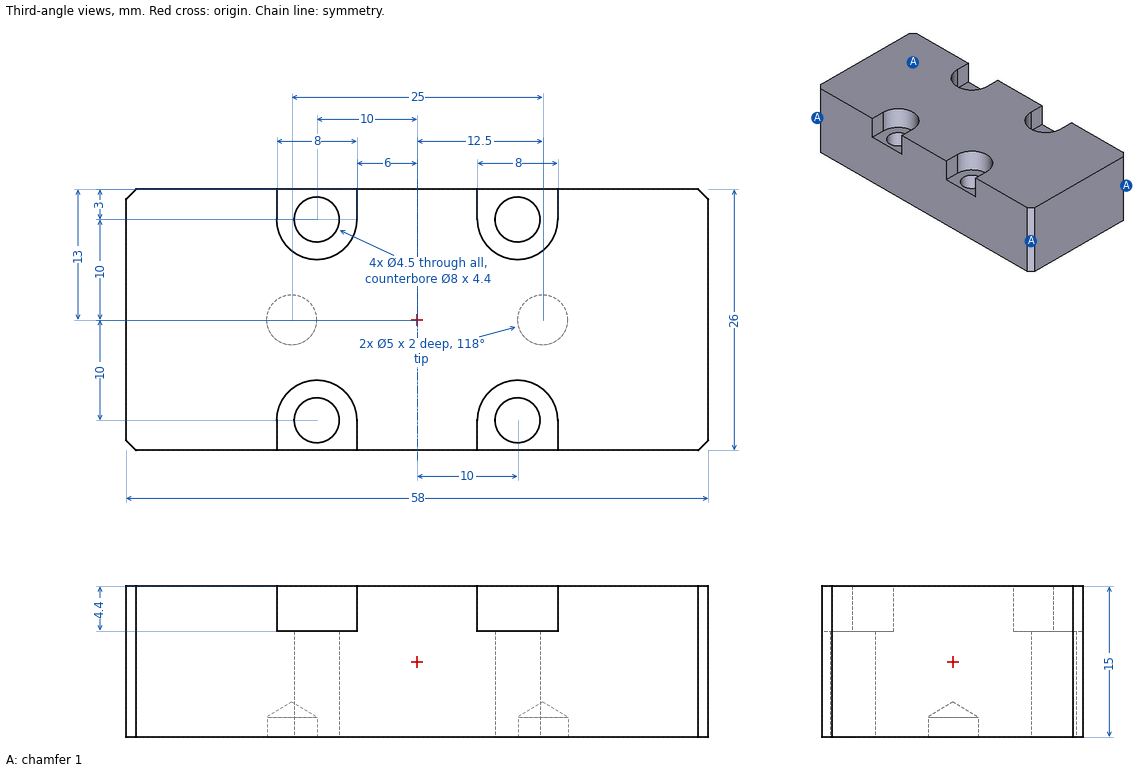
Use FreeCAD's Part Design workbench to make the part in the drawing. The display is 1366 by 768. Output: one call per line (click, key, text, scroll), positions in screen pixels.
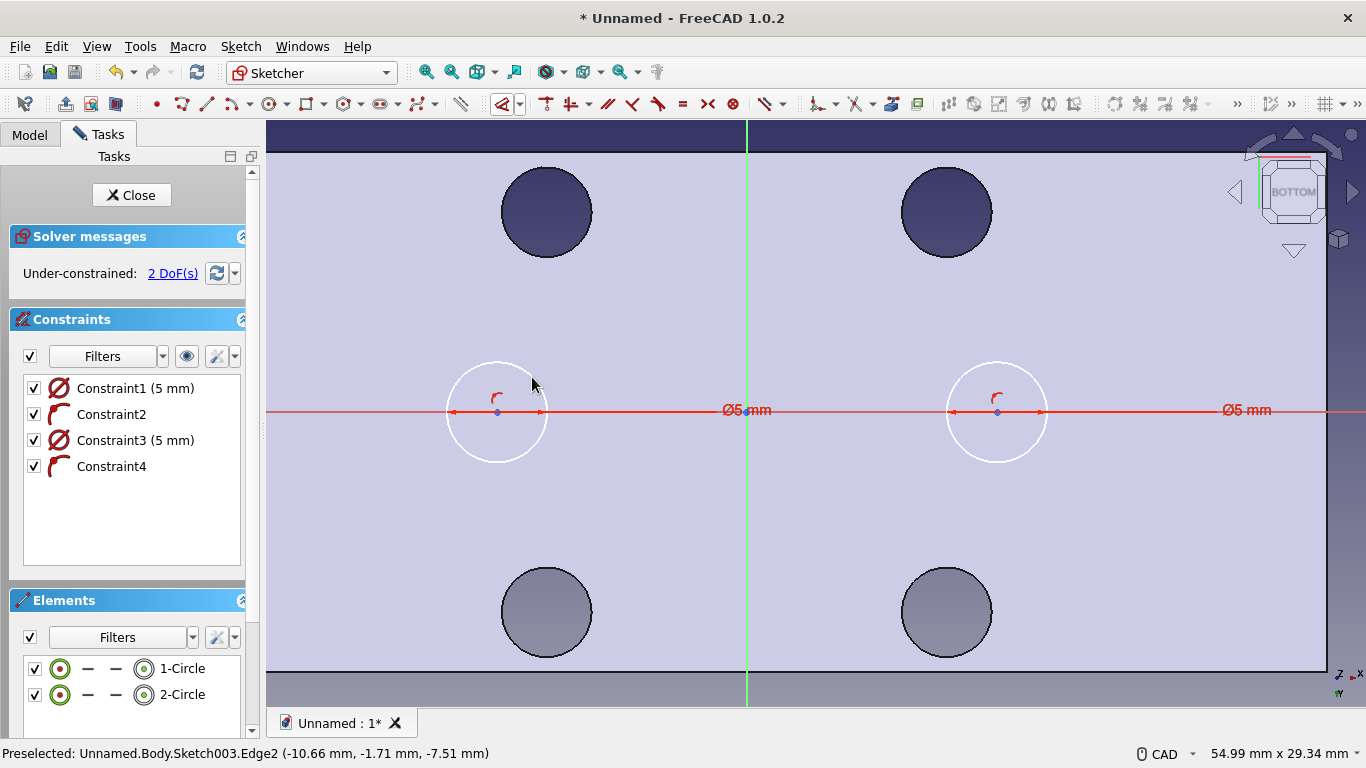
click(997, 412)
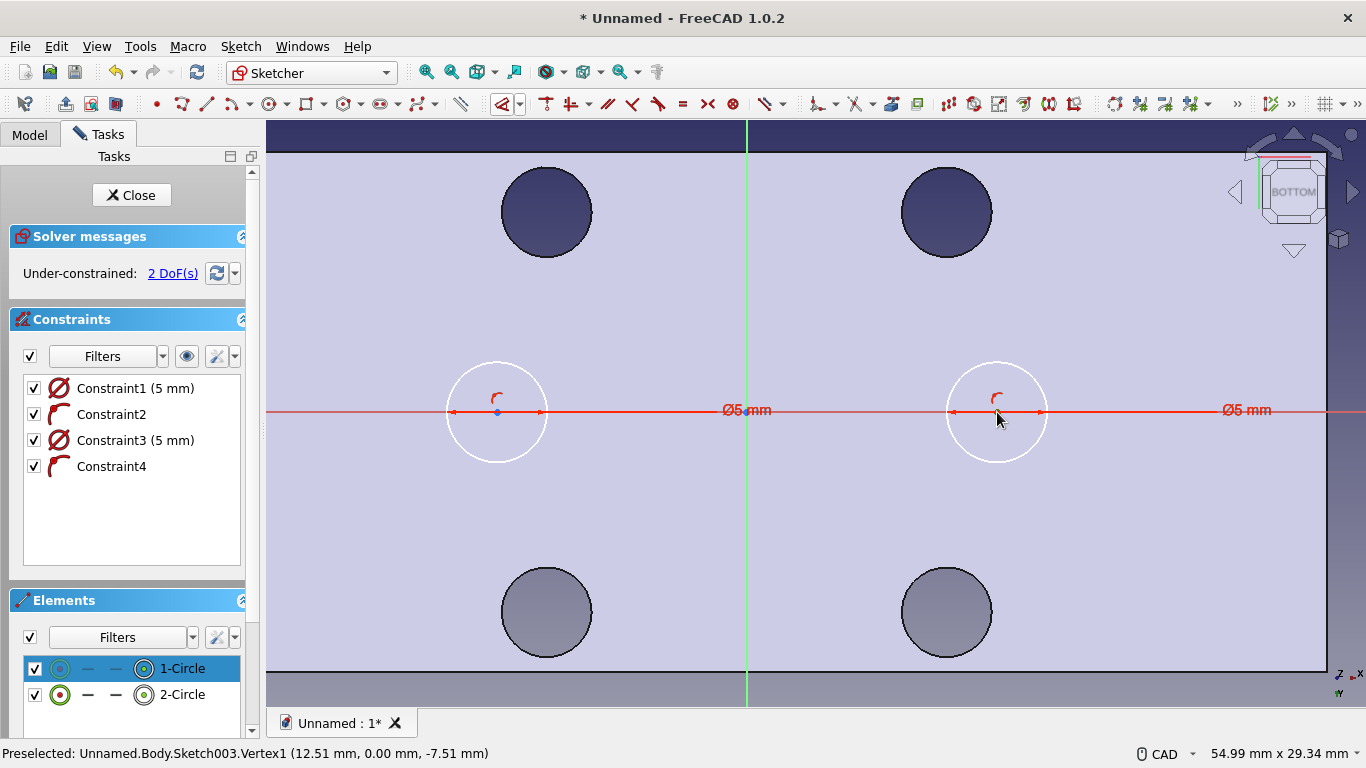
click(497, 412)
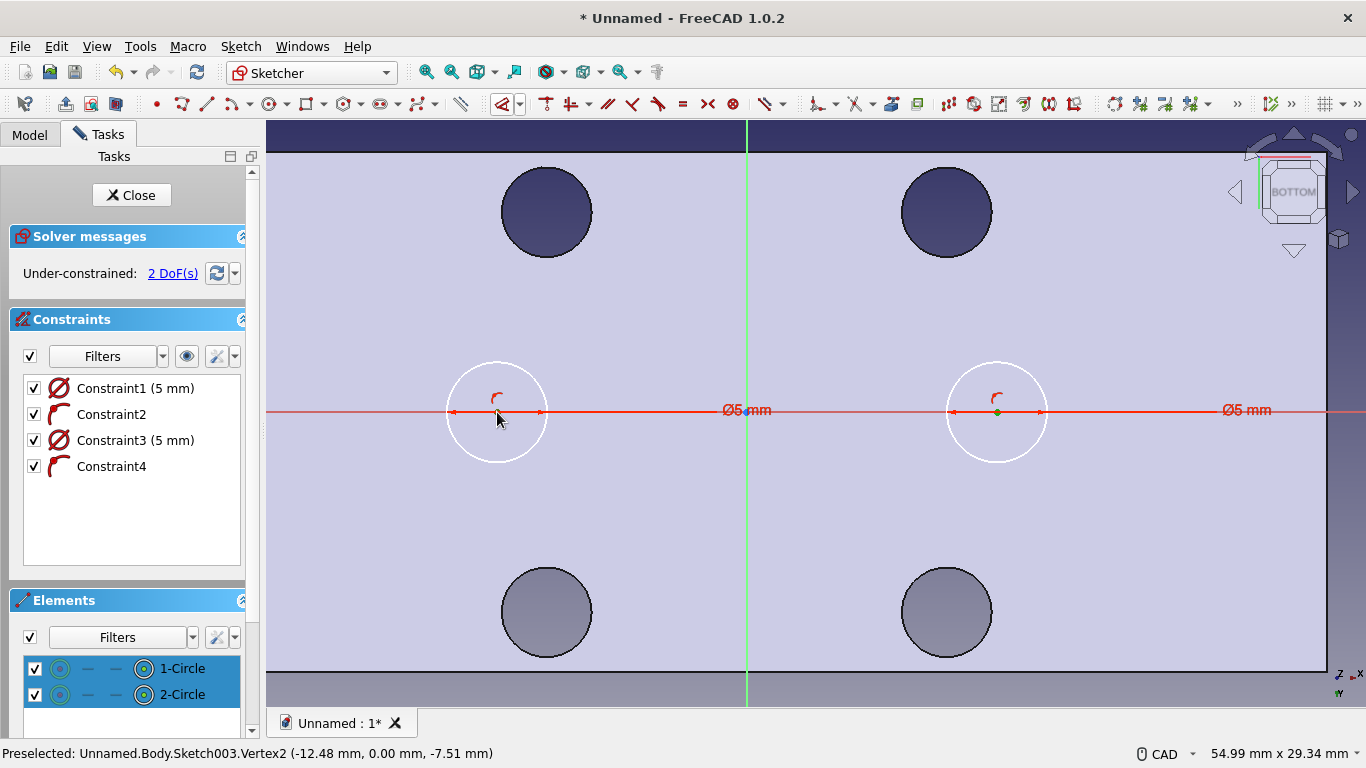
click(520, 104)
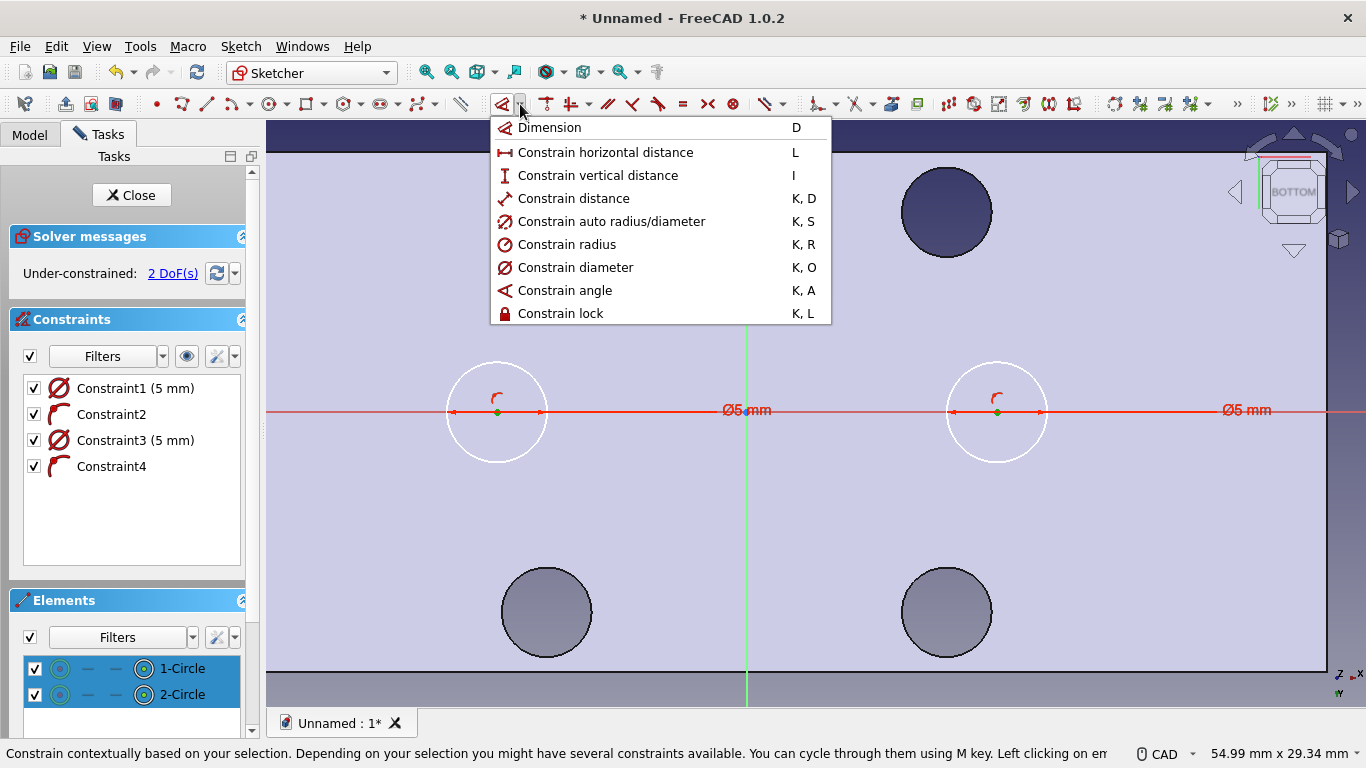
click(661, 152)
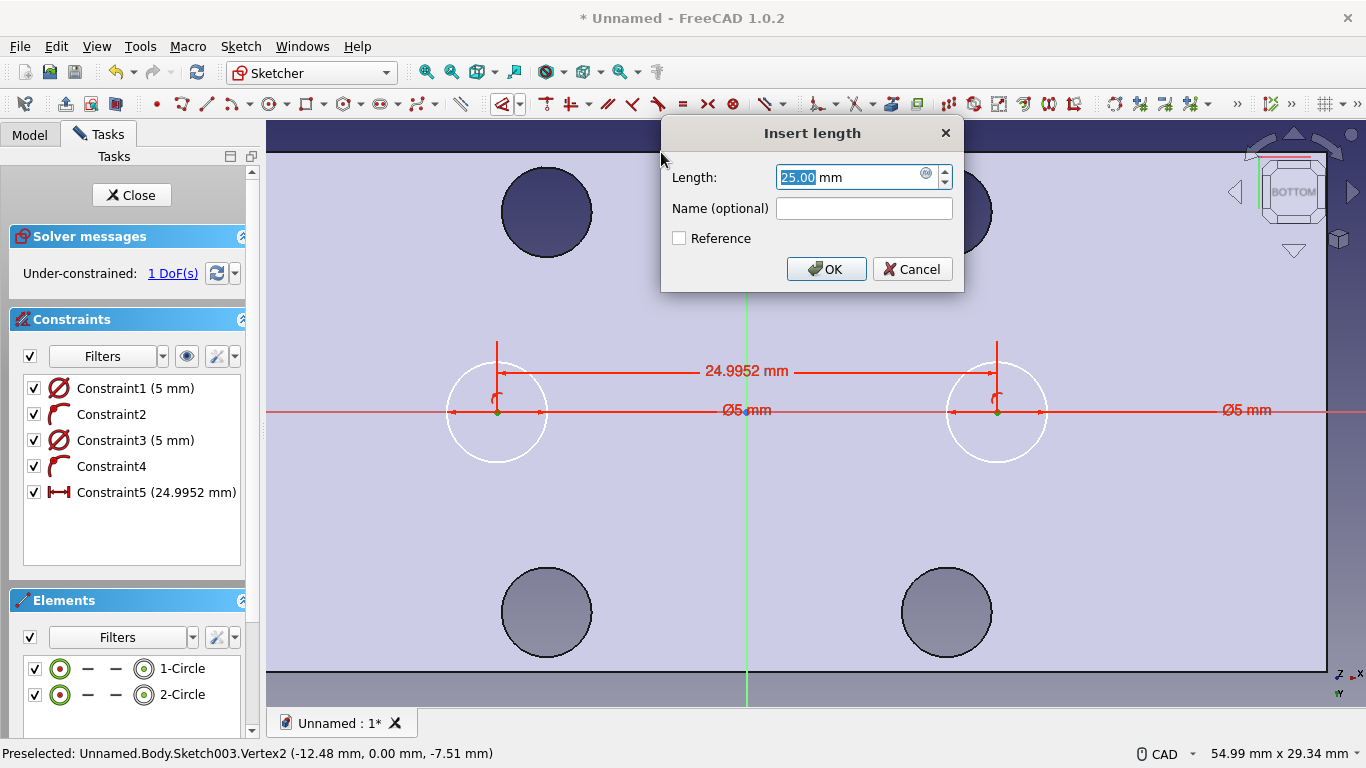
text(25)
key(Return)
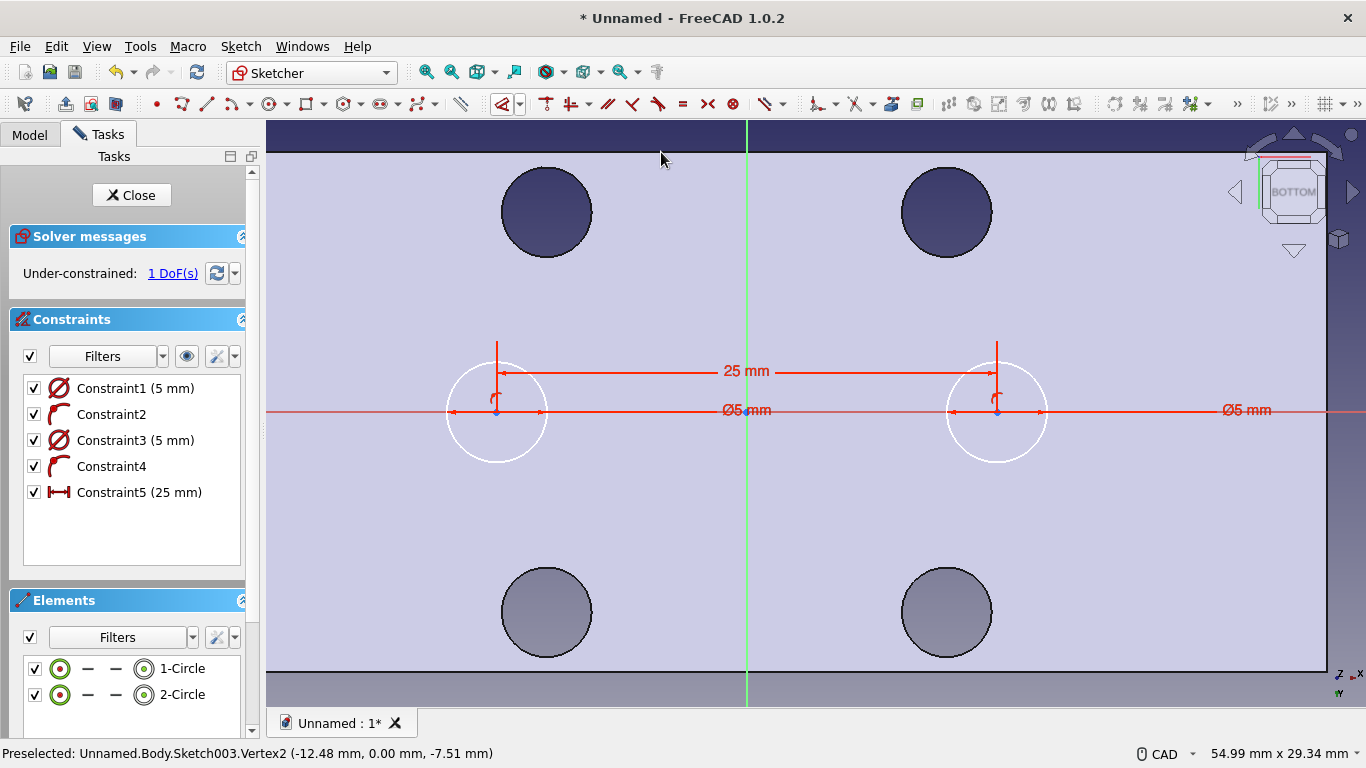
click(997, 412)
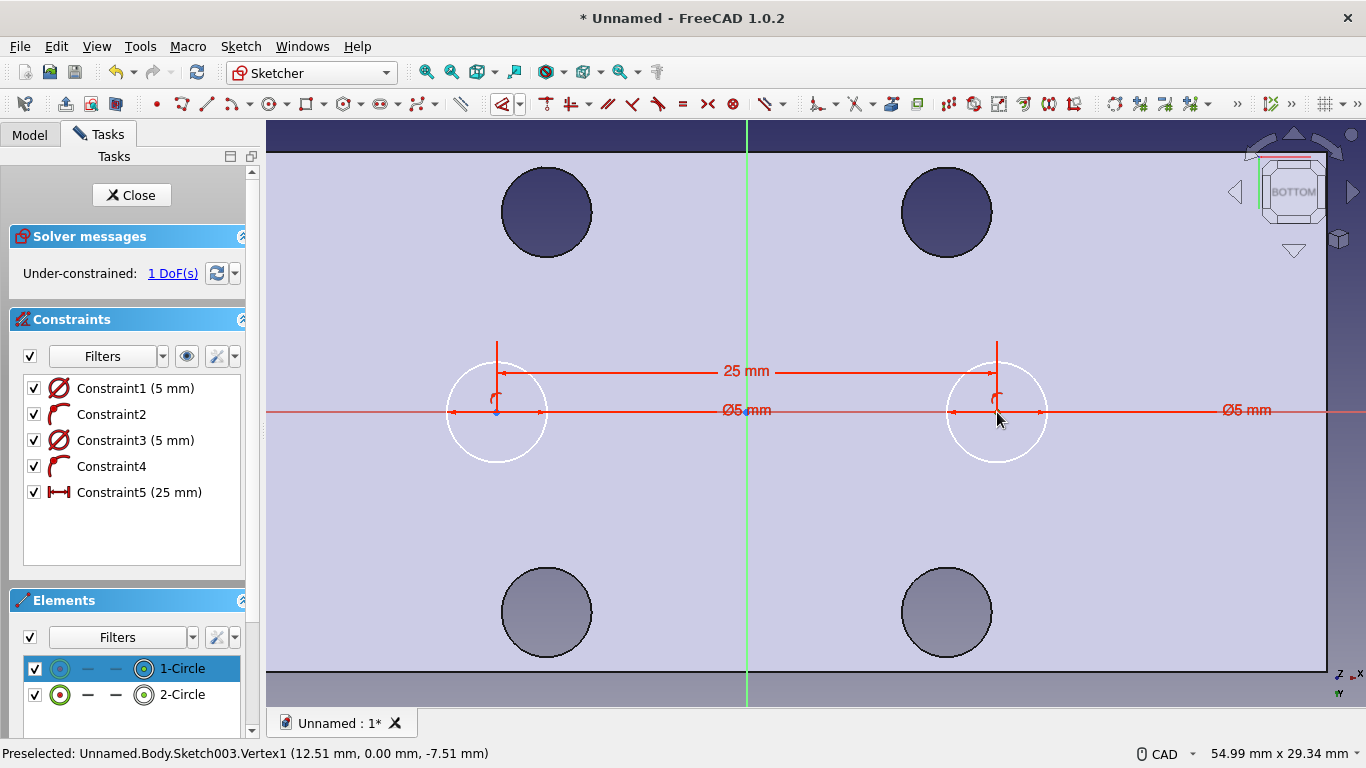
key(l)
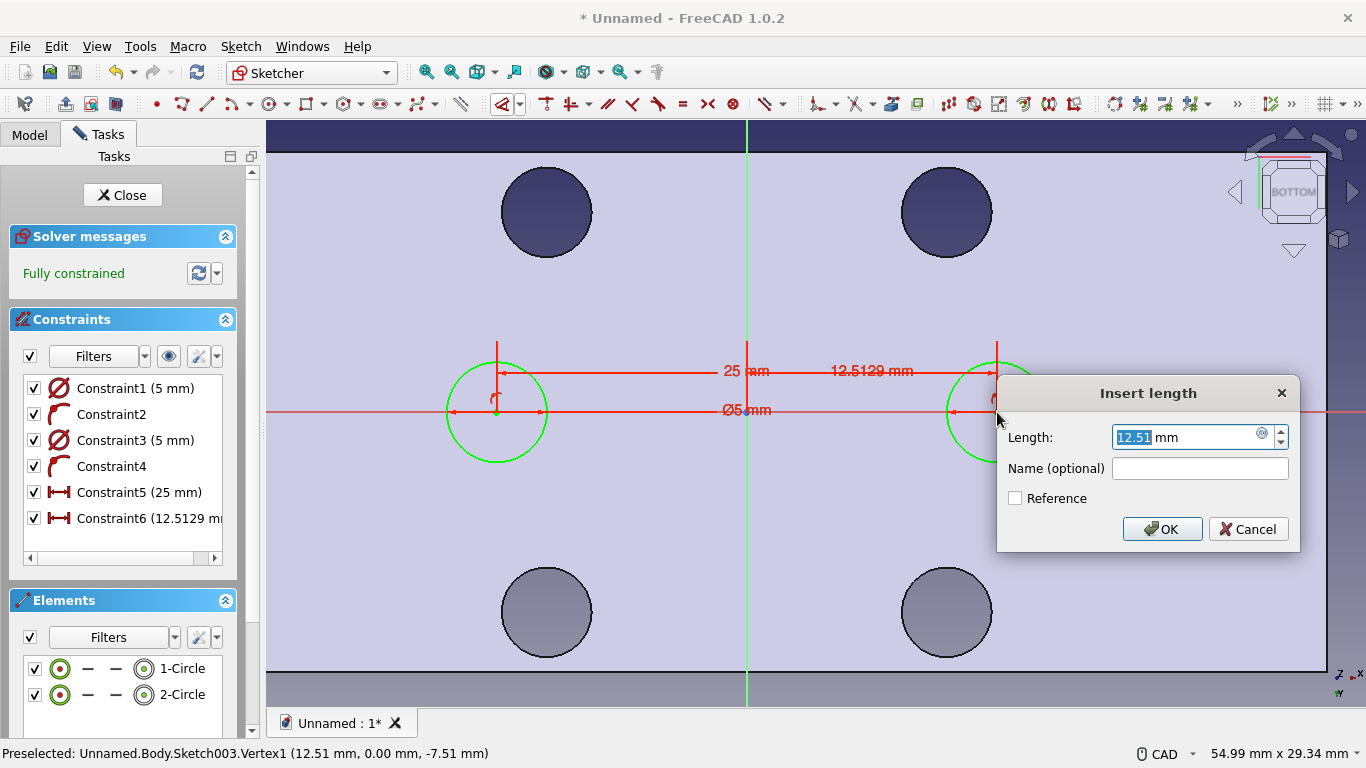
text(12.5)
key(Return)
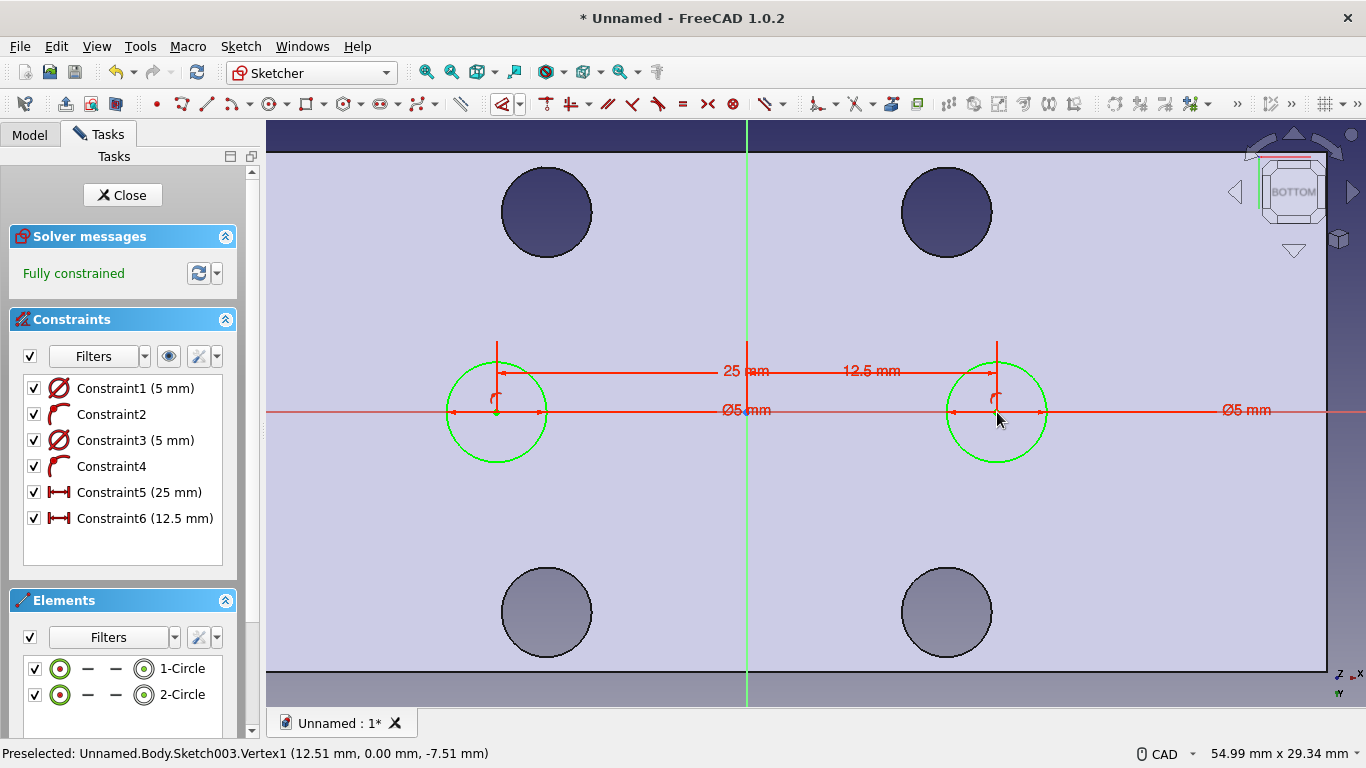
click(123, 195)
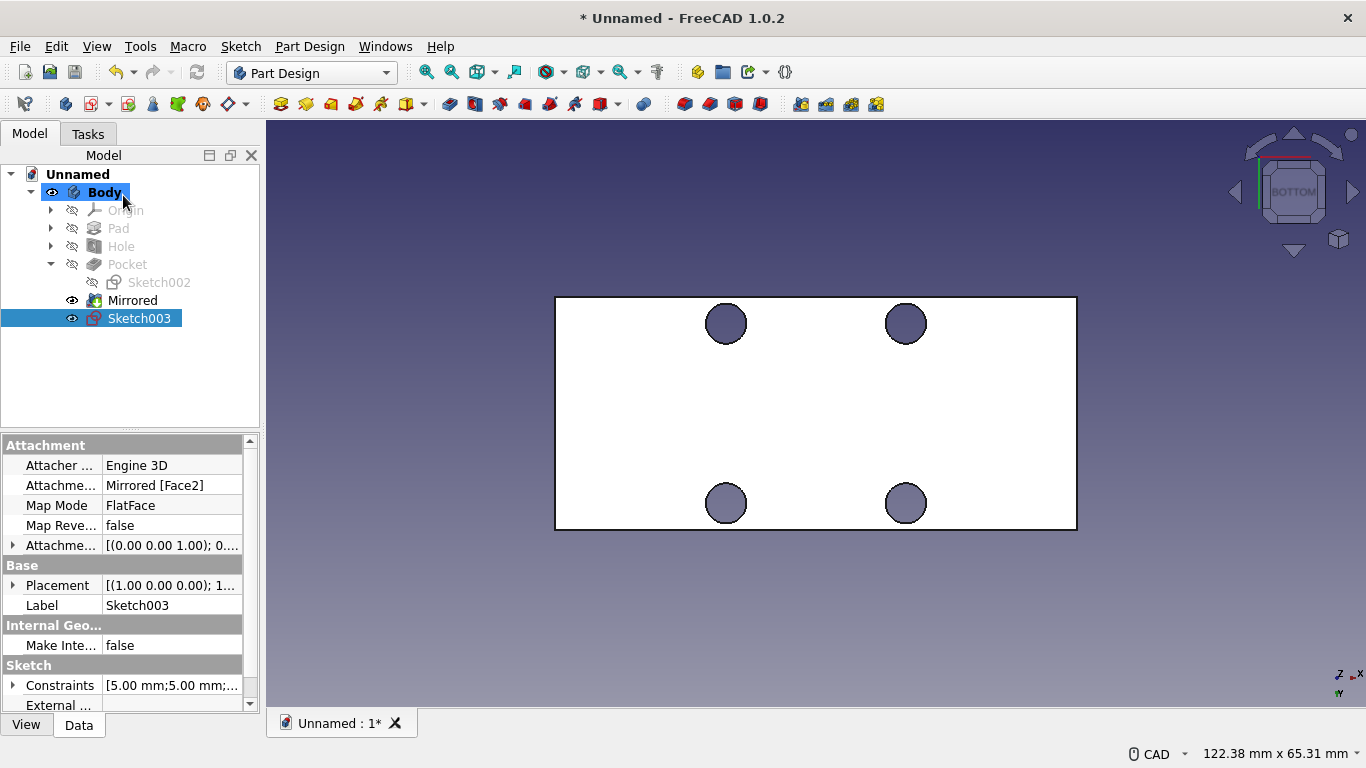
click(475, 104)